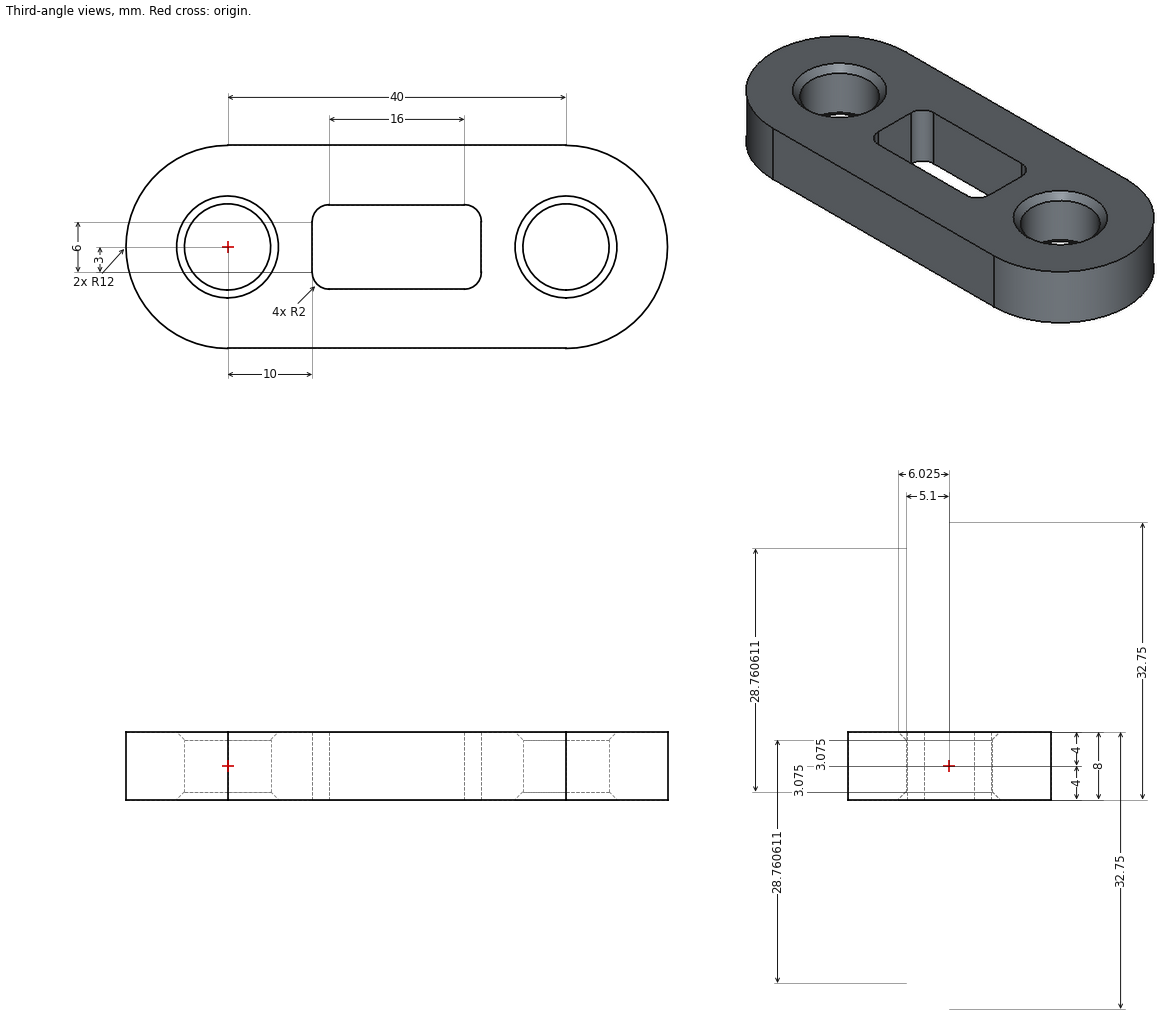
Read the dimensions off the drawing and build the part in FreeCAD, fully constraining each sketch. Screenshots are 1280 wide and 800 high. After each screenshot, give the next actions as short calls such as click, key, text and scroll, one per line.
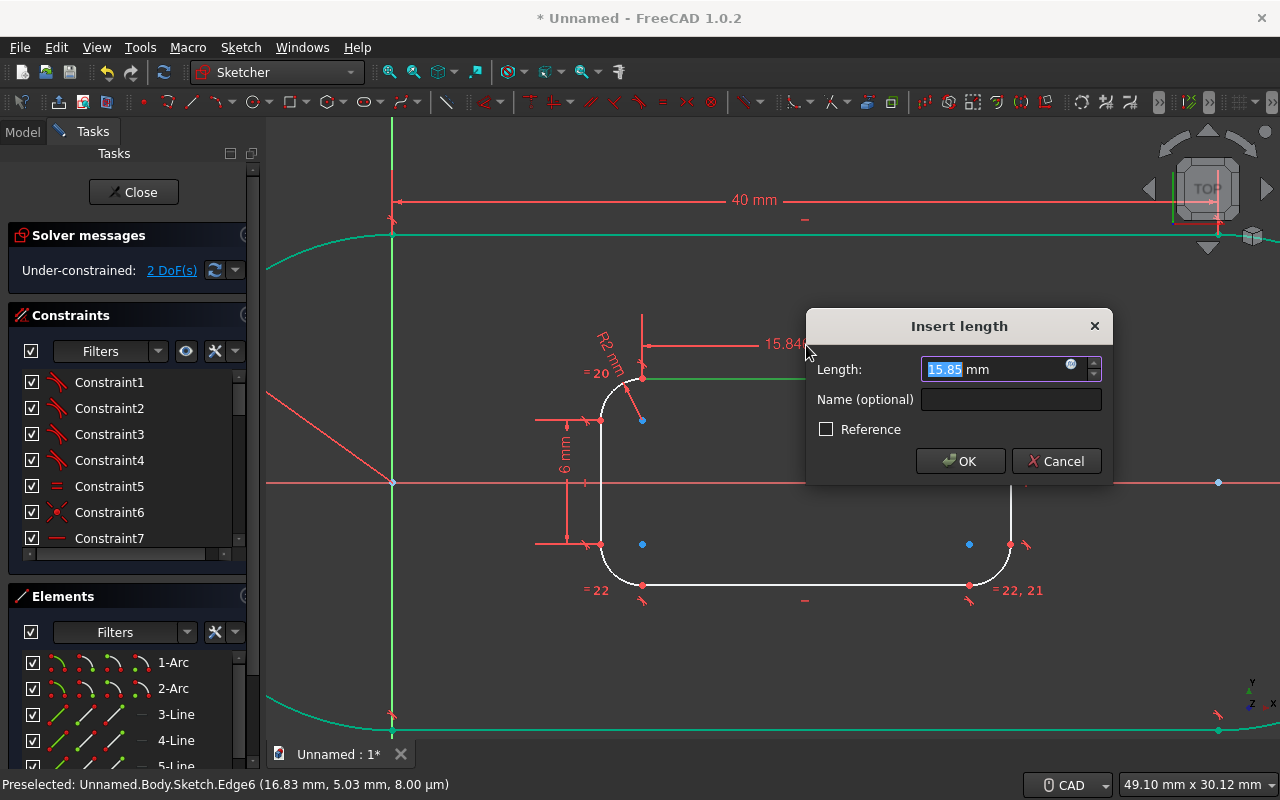
text(16)
key(Return)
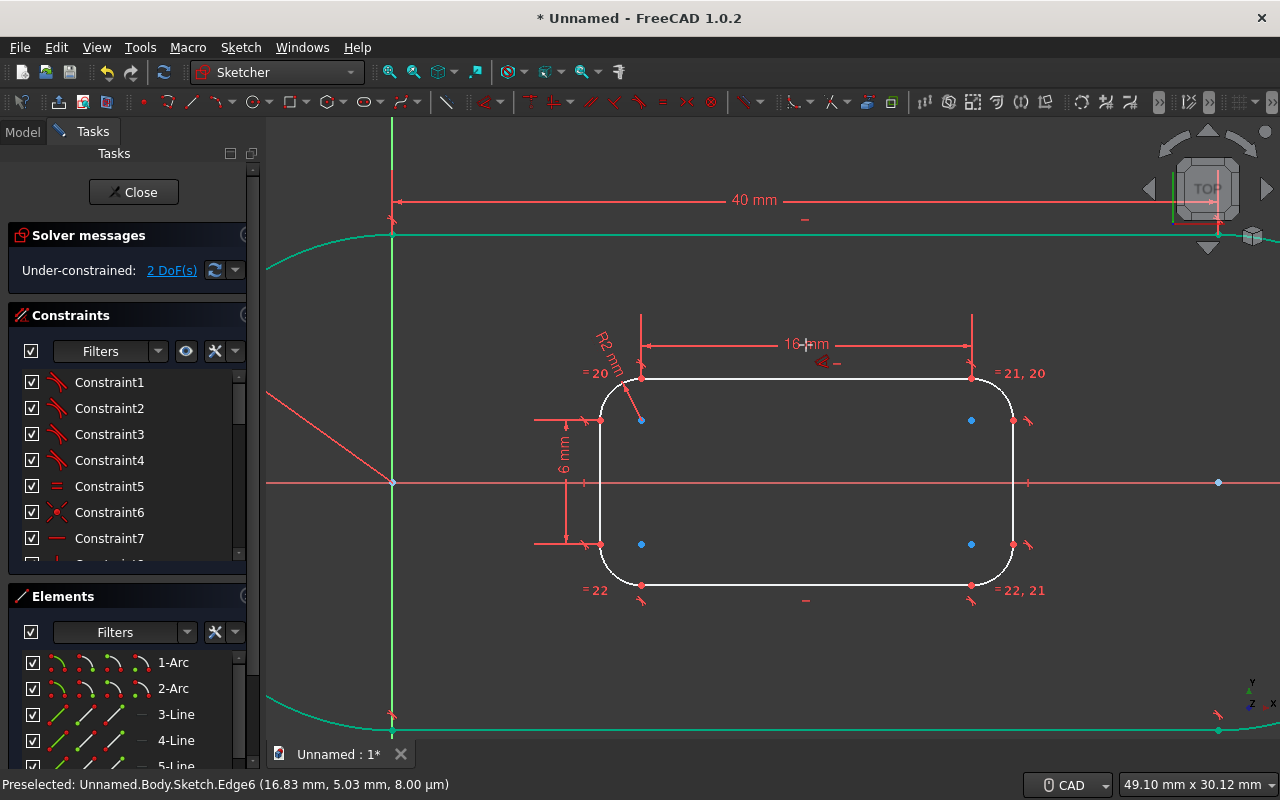
click(600, 544)
click(358, 513)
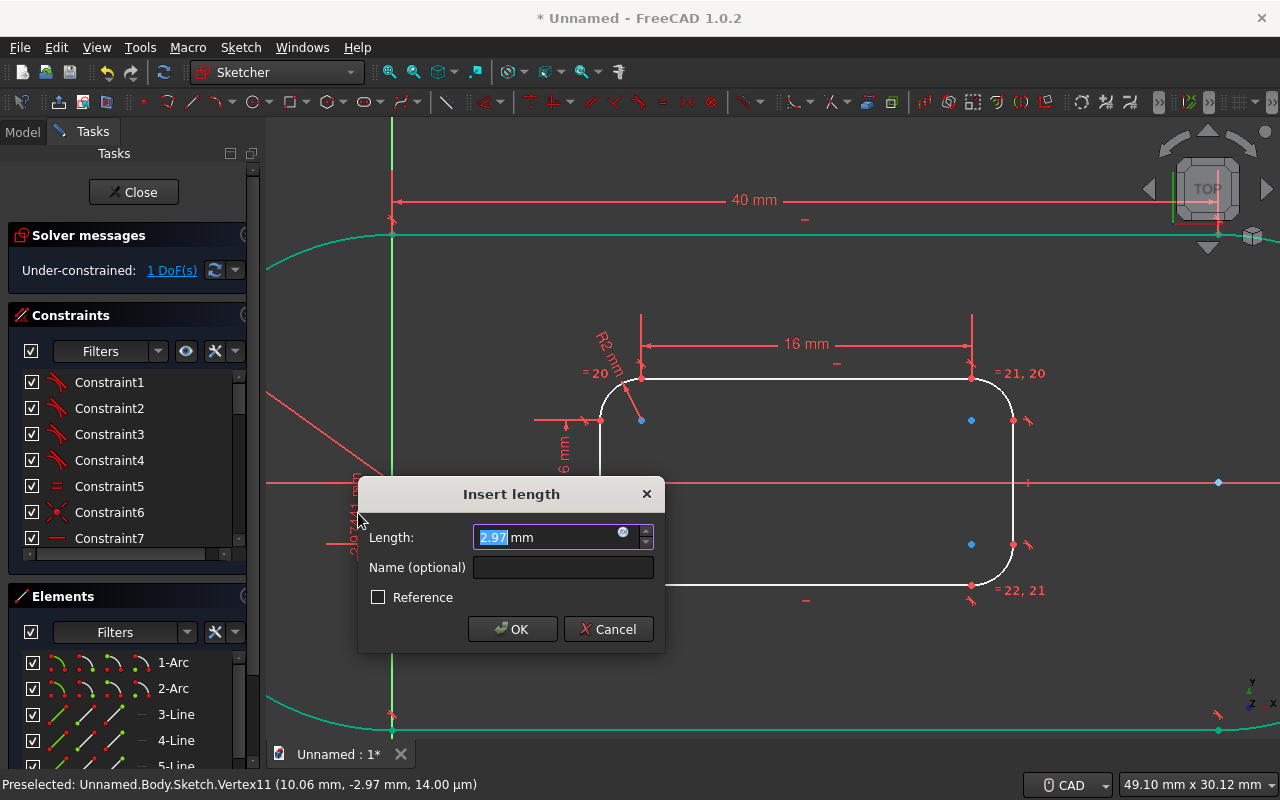
text(3)
key(Return)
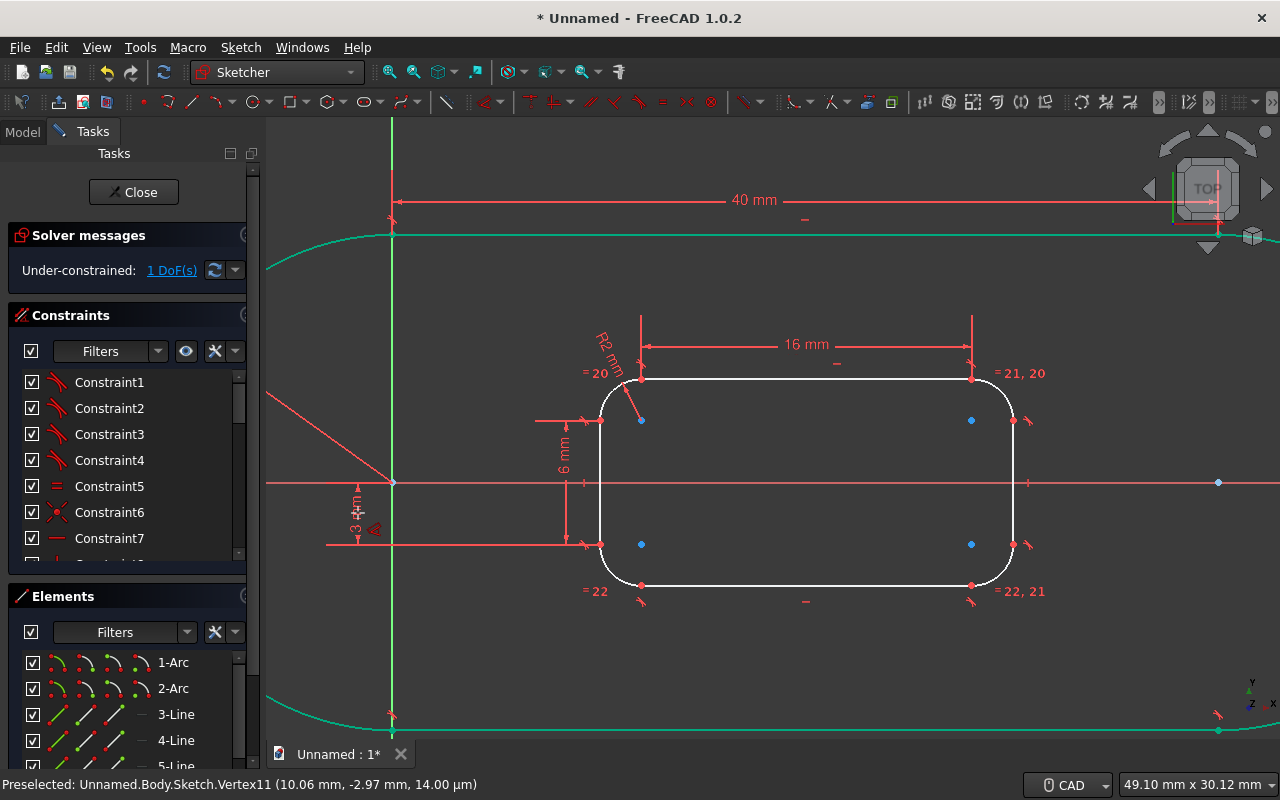
click(600, 545)
click(496, 579)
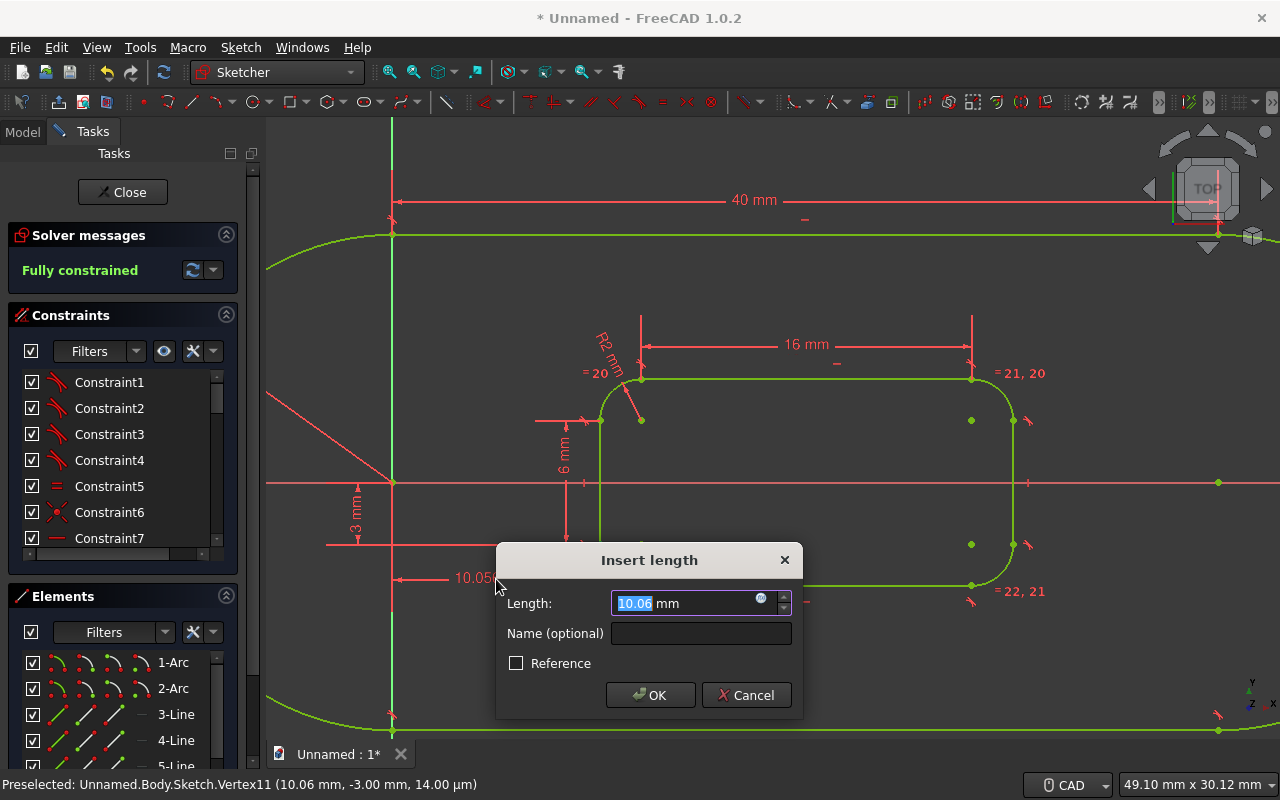
text(10)
key(Return)
key(Escape)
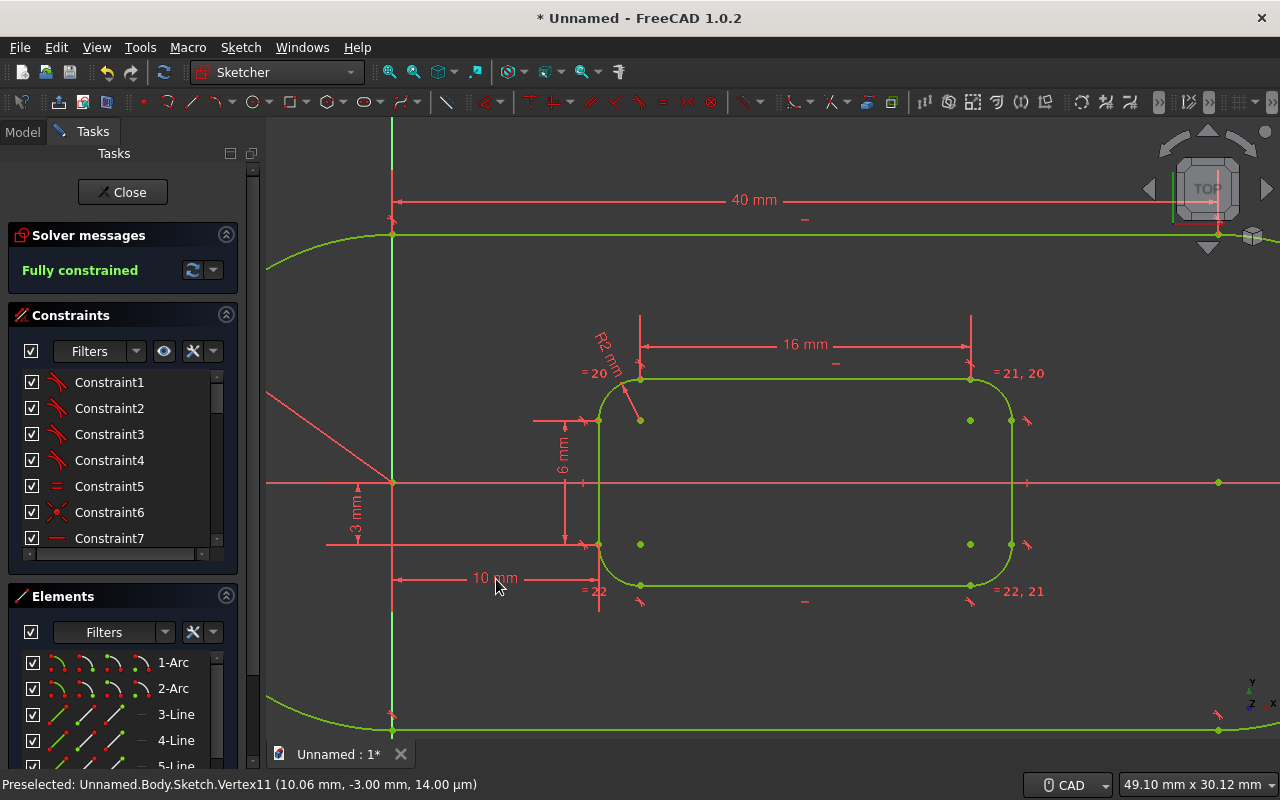
click(123, 192)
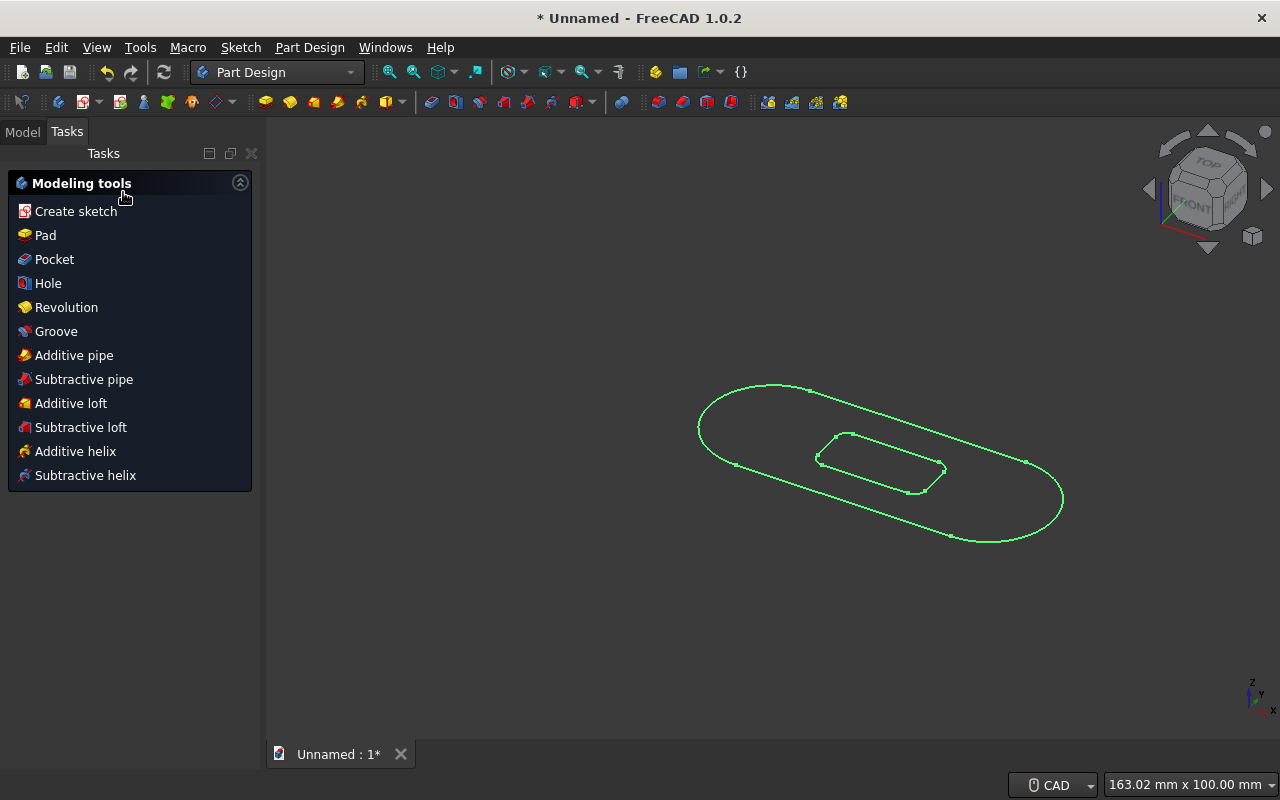
click(266, 102)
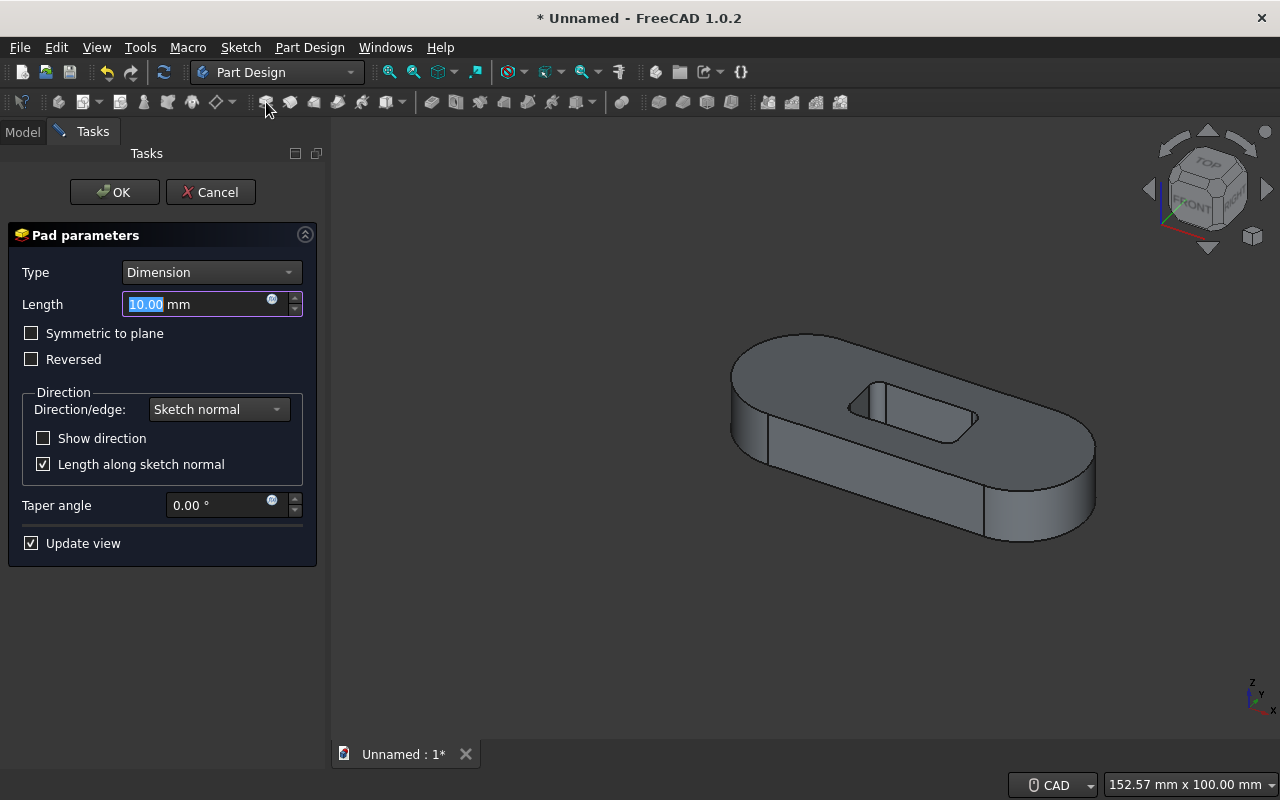
text(8)
key(Tab)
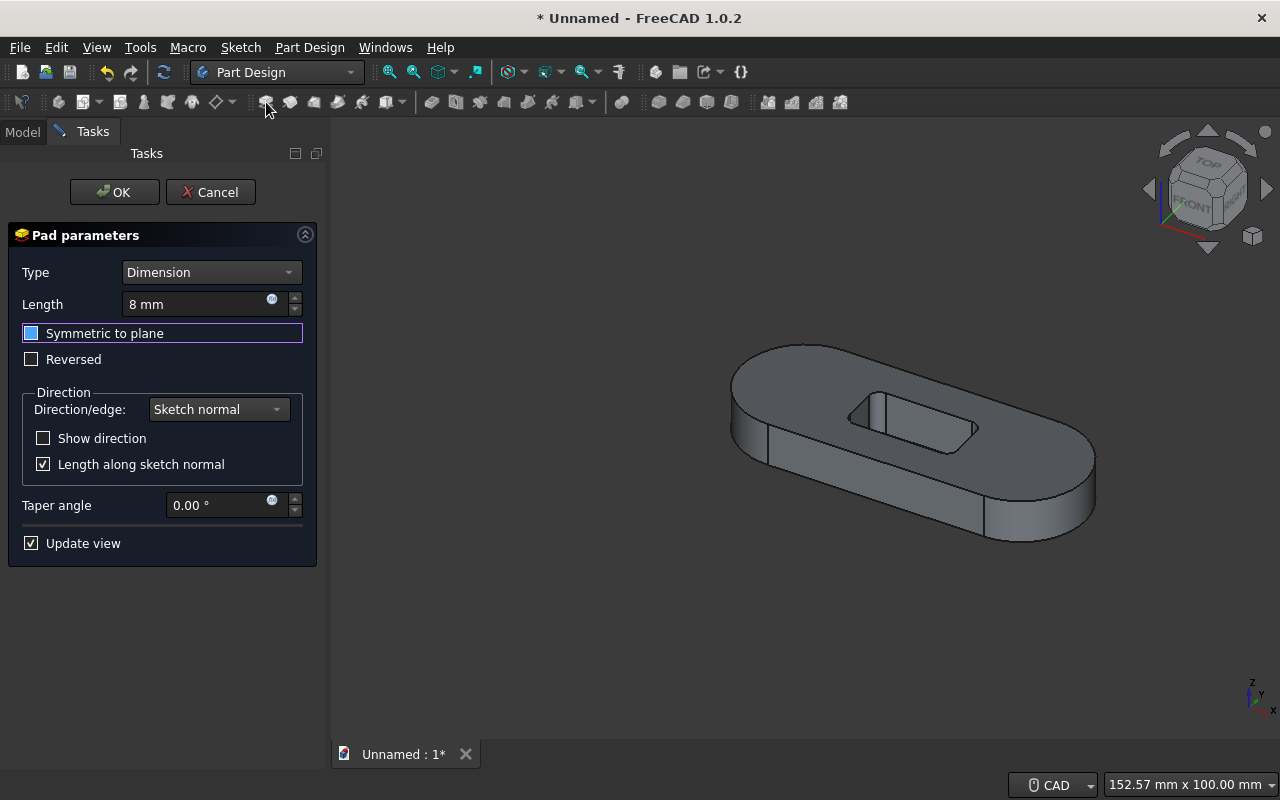
click(30, 333)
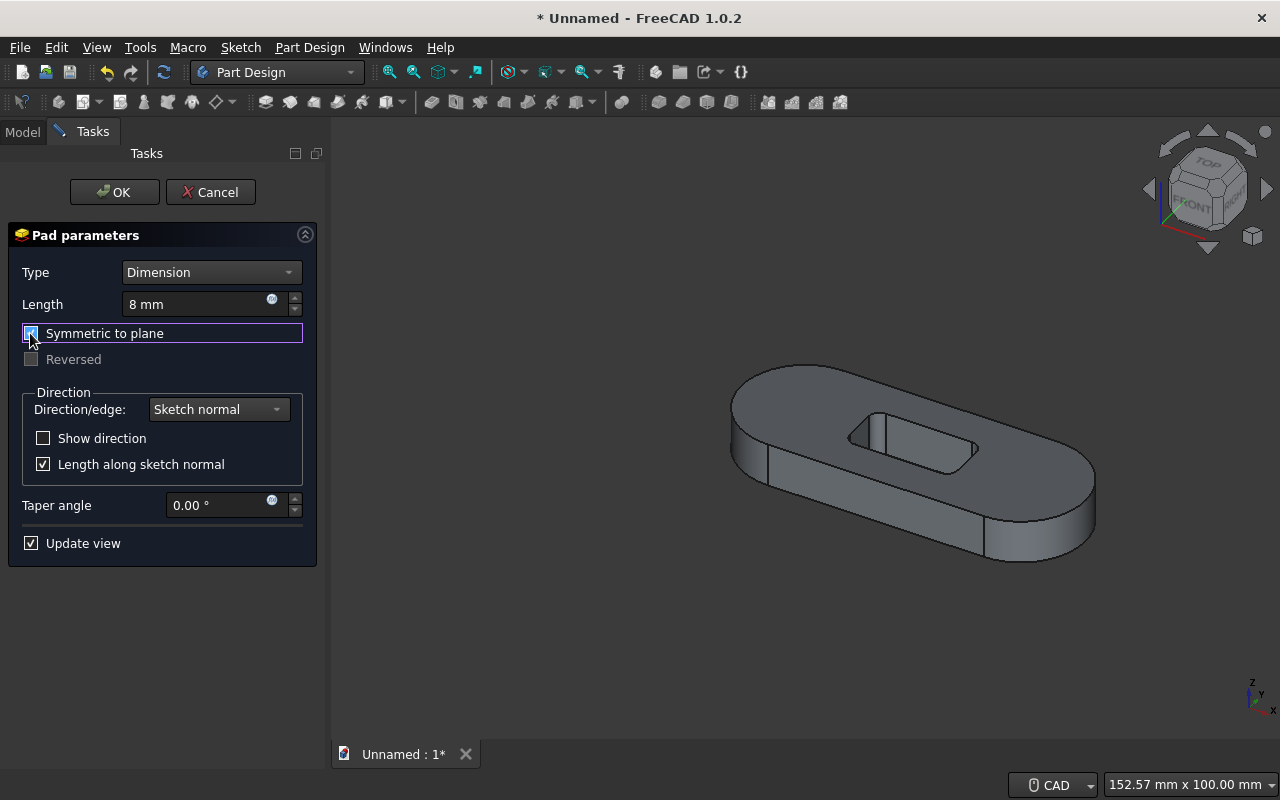
click(115, 192)